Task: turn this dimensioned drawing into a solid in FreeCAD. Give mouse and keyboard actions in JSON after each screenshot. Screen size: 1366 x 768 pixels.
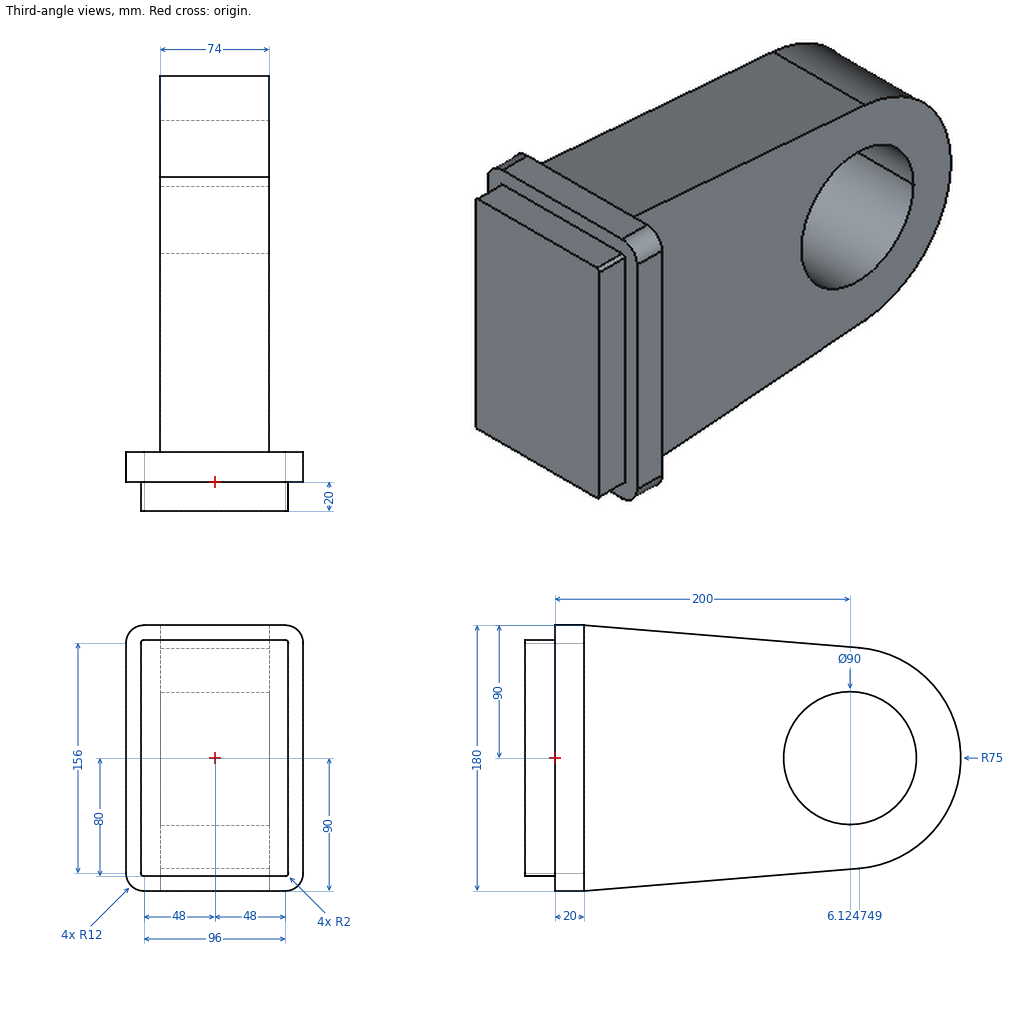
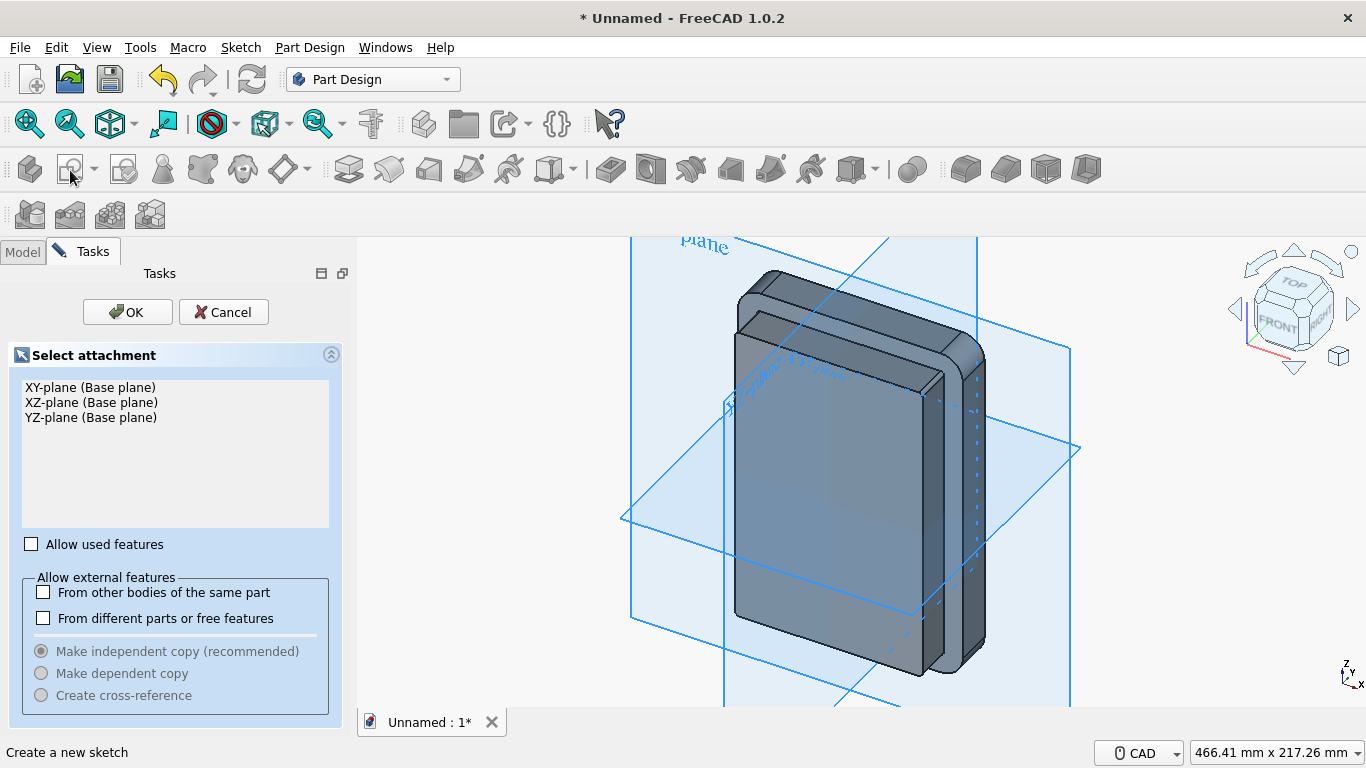
{"action": "left_click", "coordinate": [82, 418]}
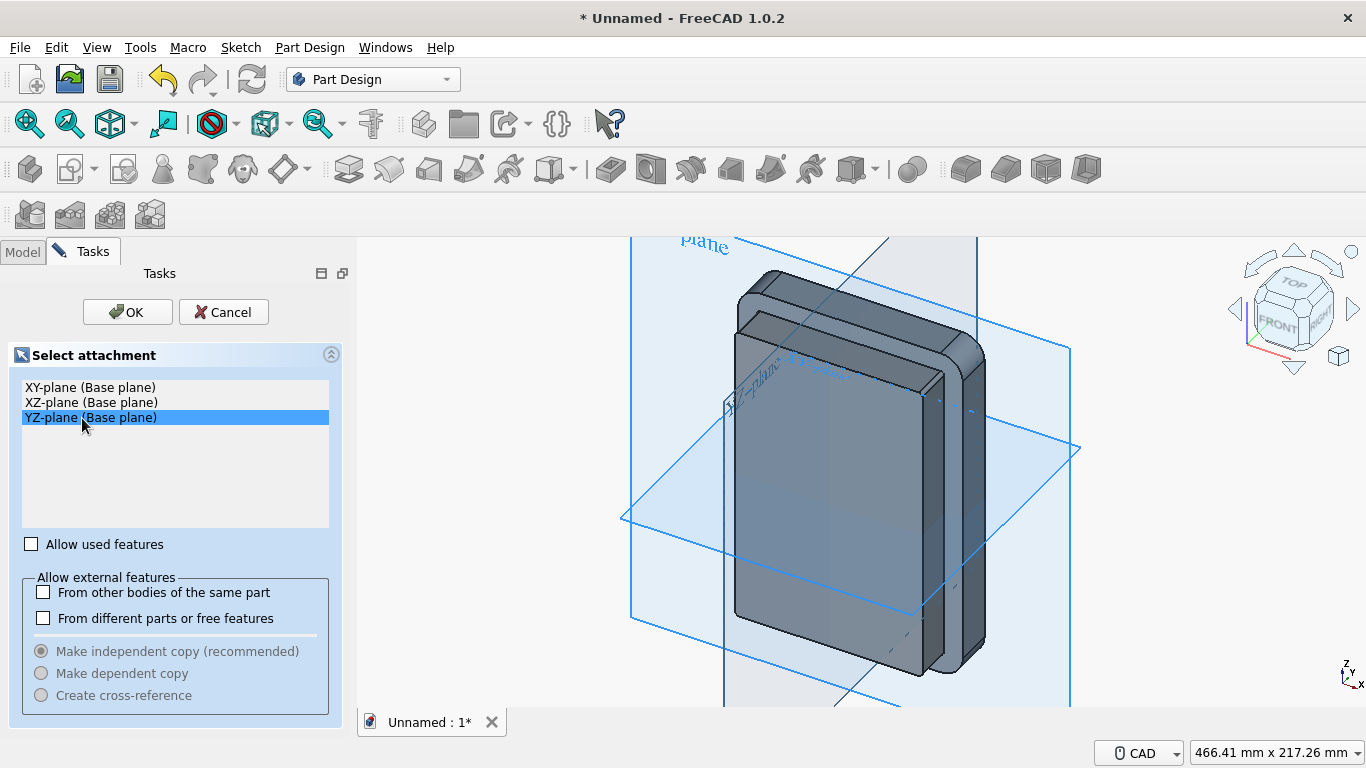
{"action": "left_click", "coordinate": [128, 312]}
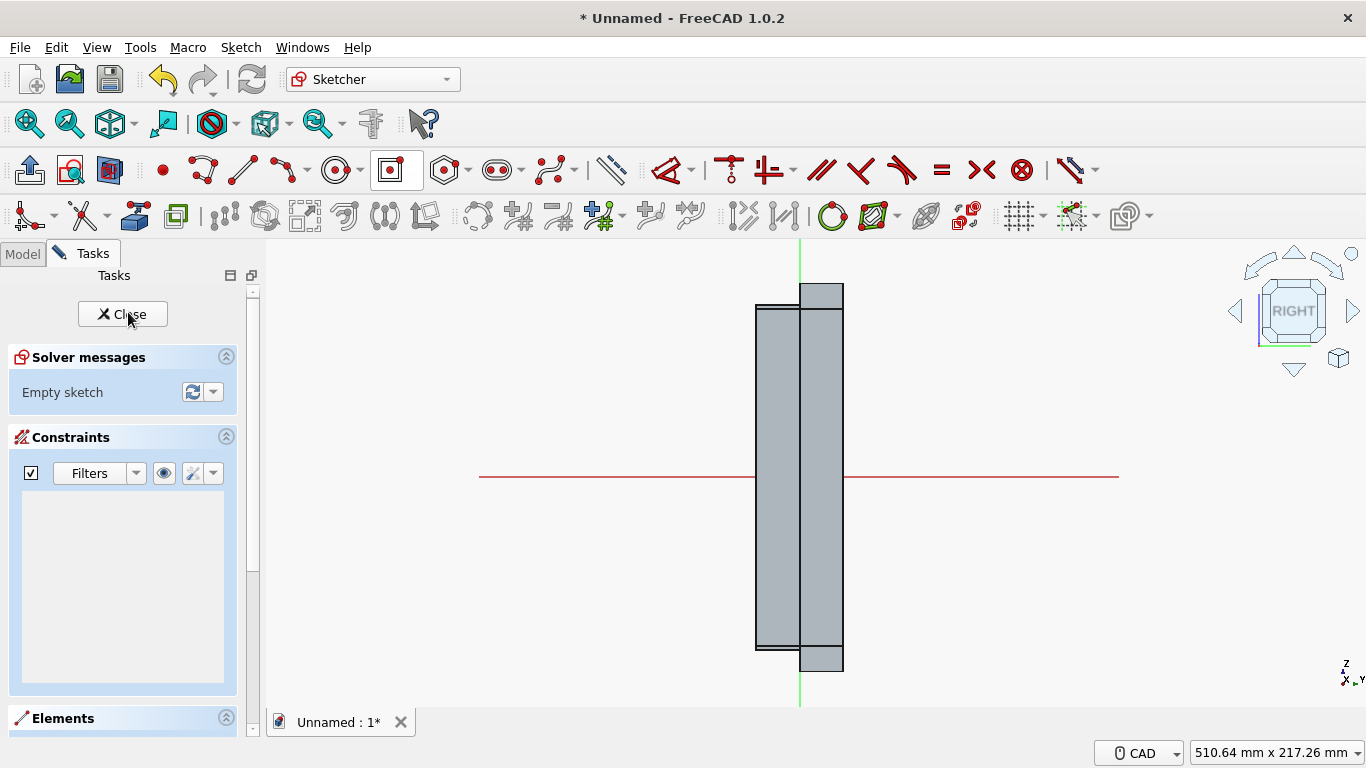
{"action": "key", "text": "q s"}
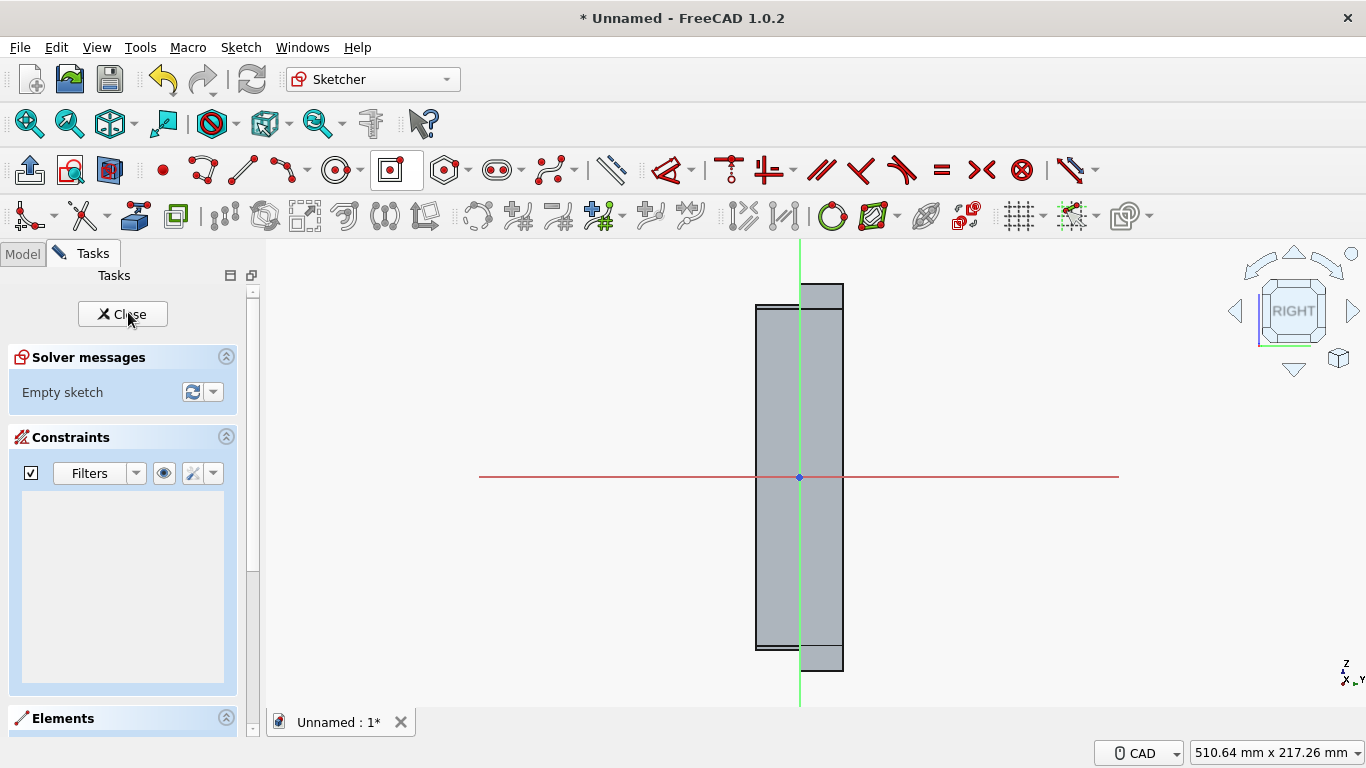
{"action": "scroll", "coordinate": [294, 464], "scroll_direction": "down", "scroll_amount": 2}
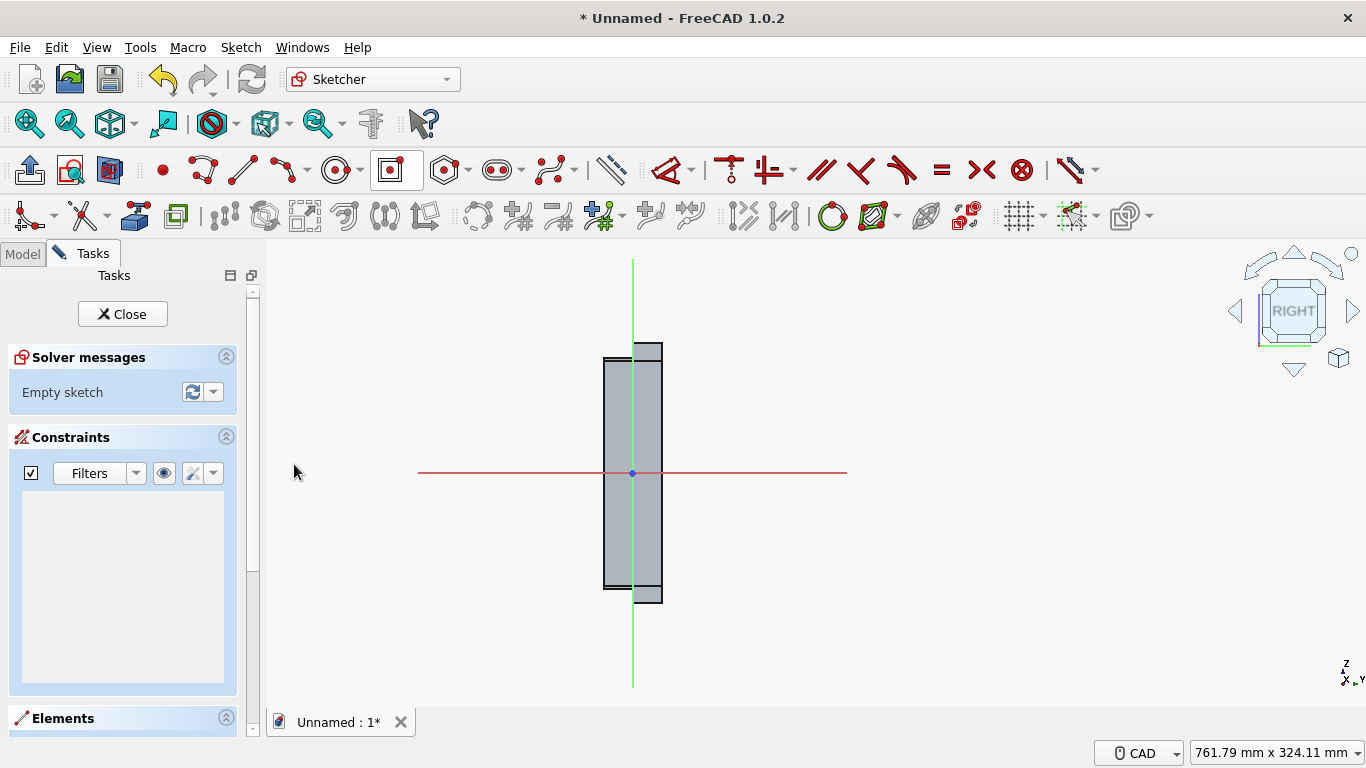
{"action": "key", "text": "g m"}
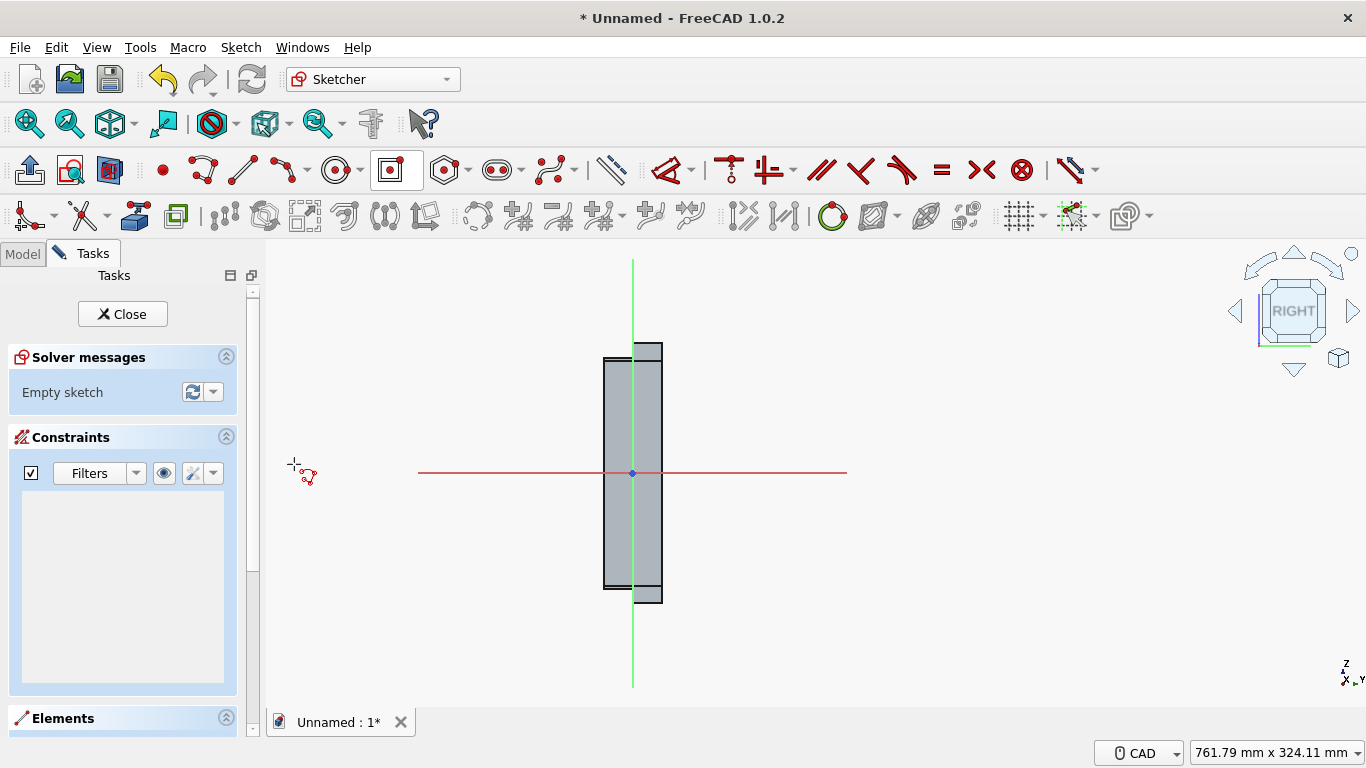
{"action": "left_click", "coordinate": [931, 365]}
{"action": "left_click", "coordinate": [662, 343]}
{"action": "left_click", "coordinate": [662, 603]}
{"action": "left_click", "coordinate": [931, 581]}
{"action": "right_click", "coordinate": [931, 581]}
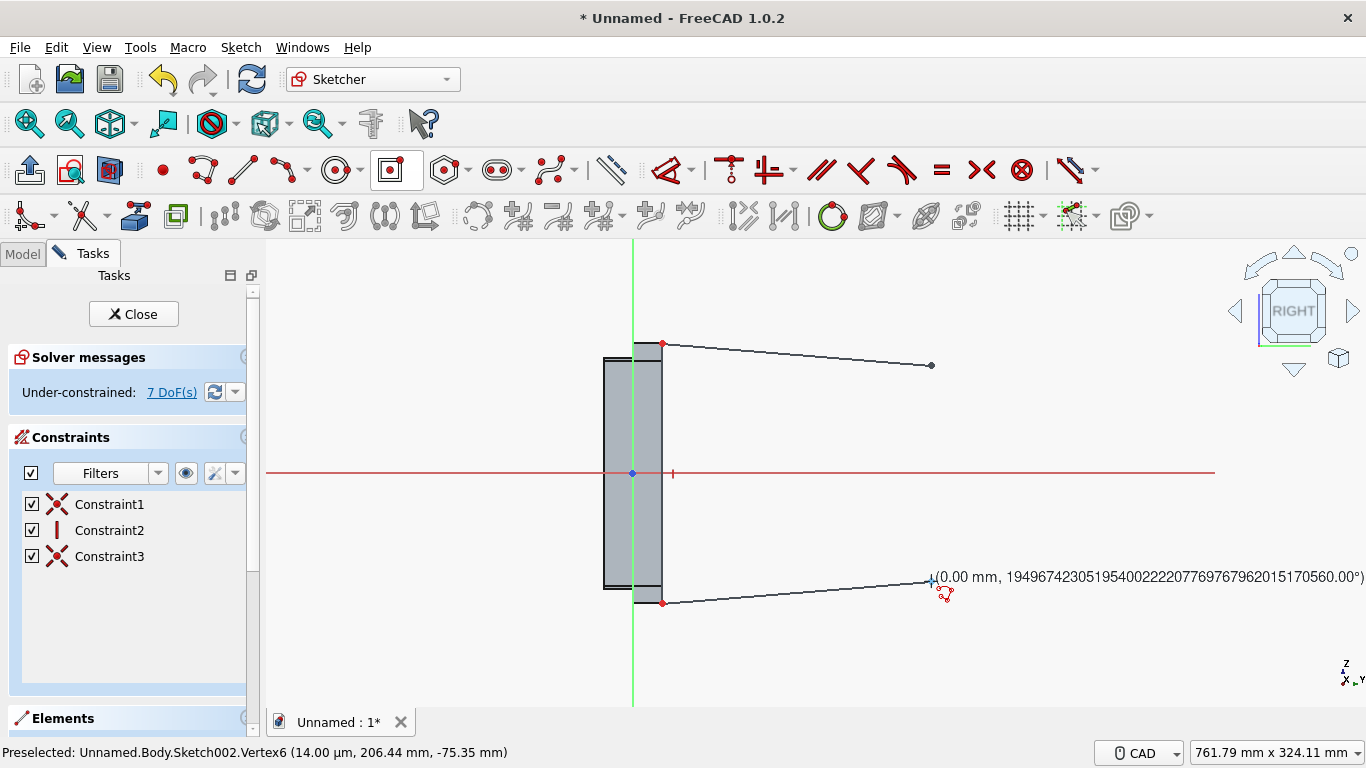
{"action": "key", "text": "g 3 a"}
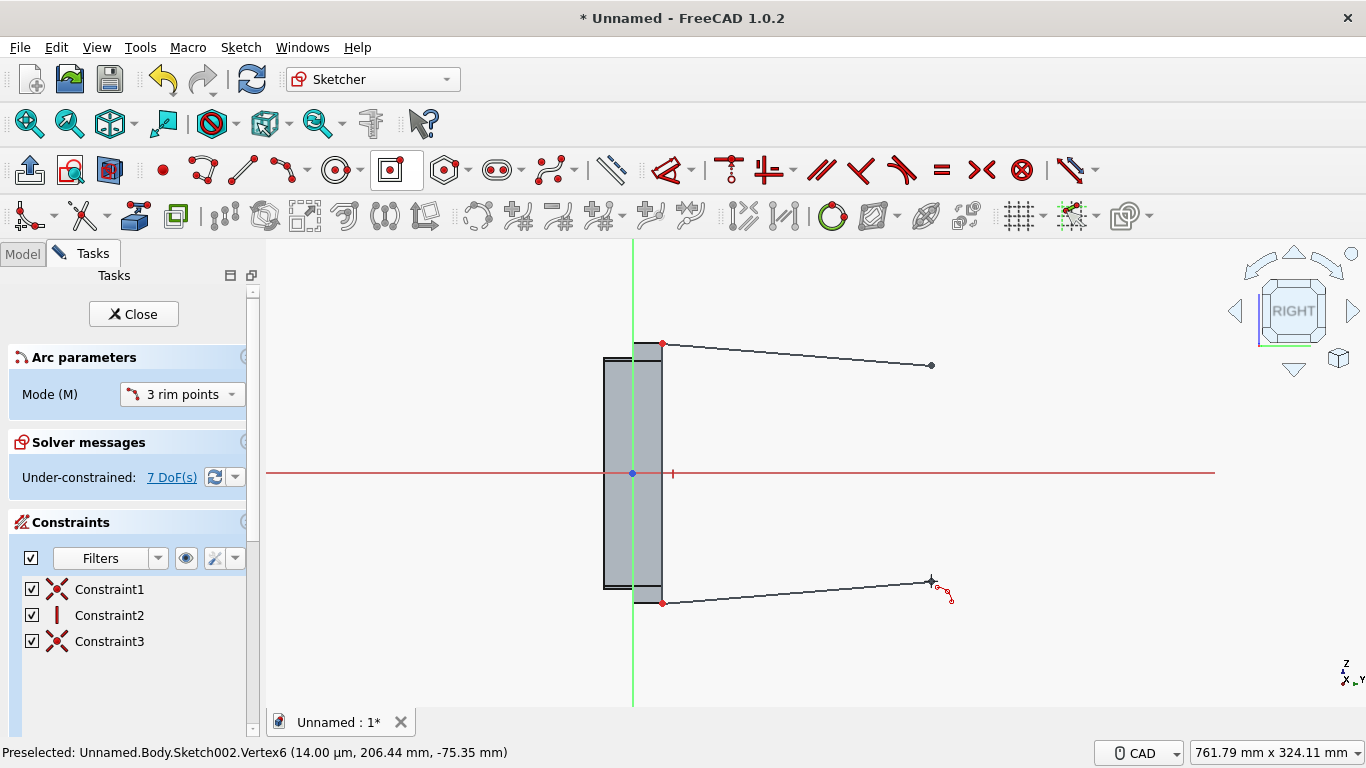
{"action": "left_click", "coordinate": [931, 582]}
{"action": "left_click", "coordinate": [931, 366]}
{"action": "left_click", "coordinate": [1025, 505]}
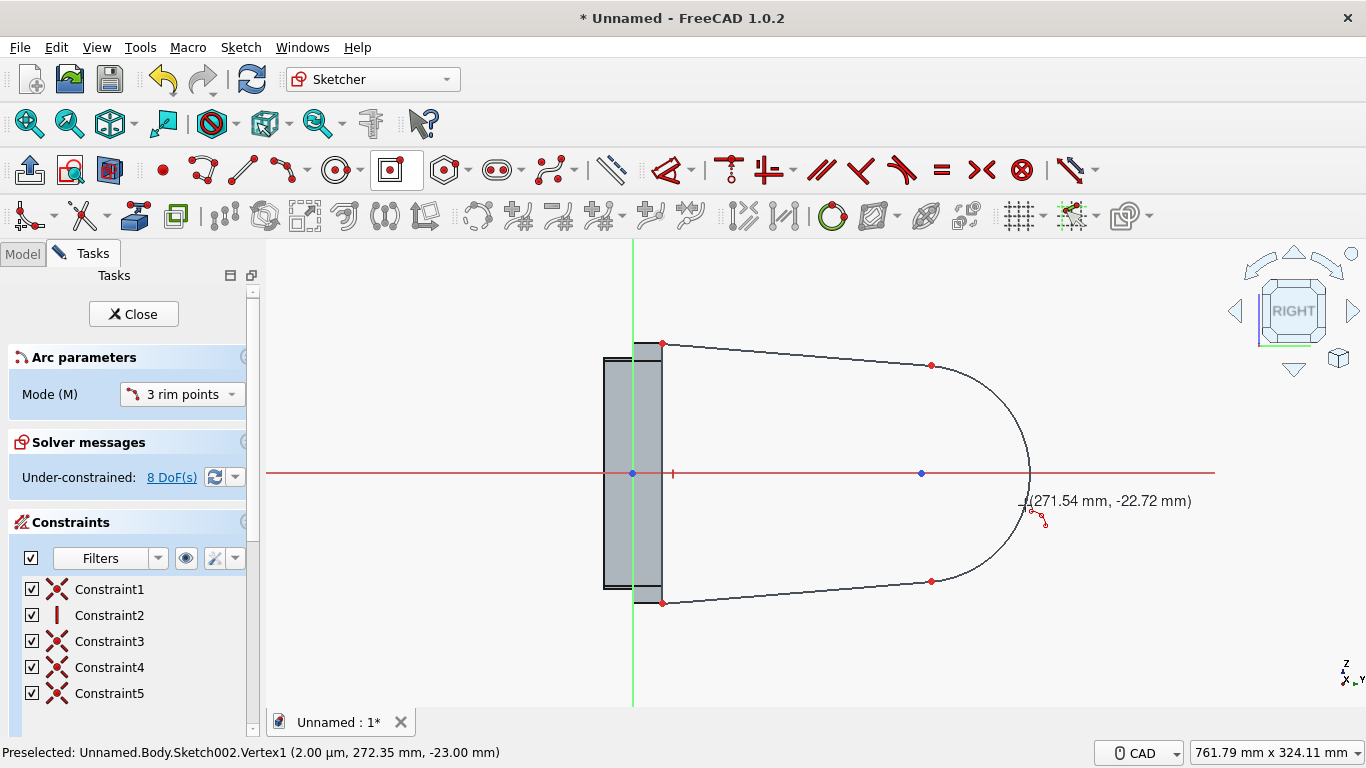
{"action": "key", "text": "g c"}